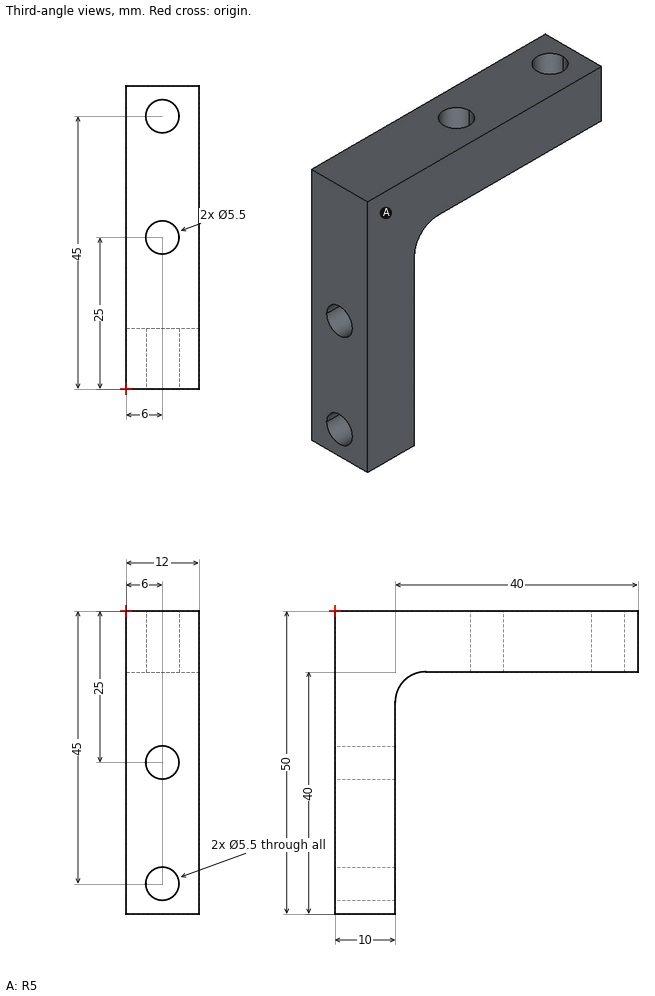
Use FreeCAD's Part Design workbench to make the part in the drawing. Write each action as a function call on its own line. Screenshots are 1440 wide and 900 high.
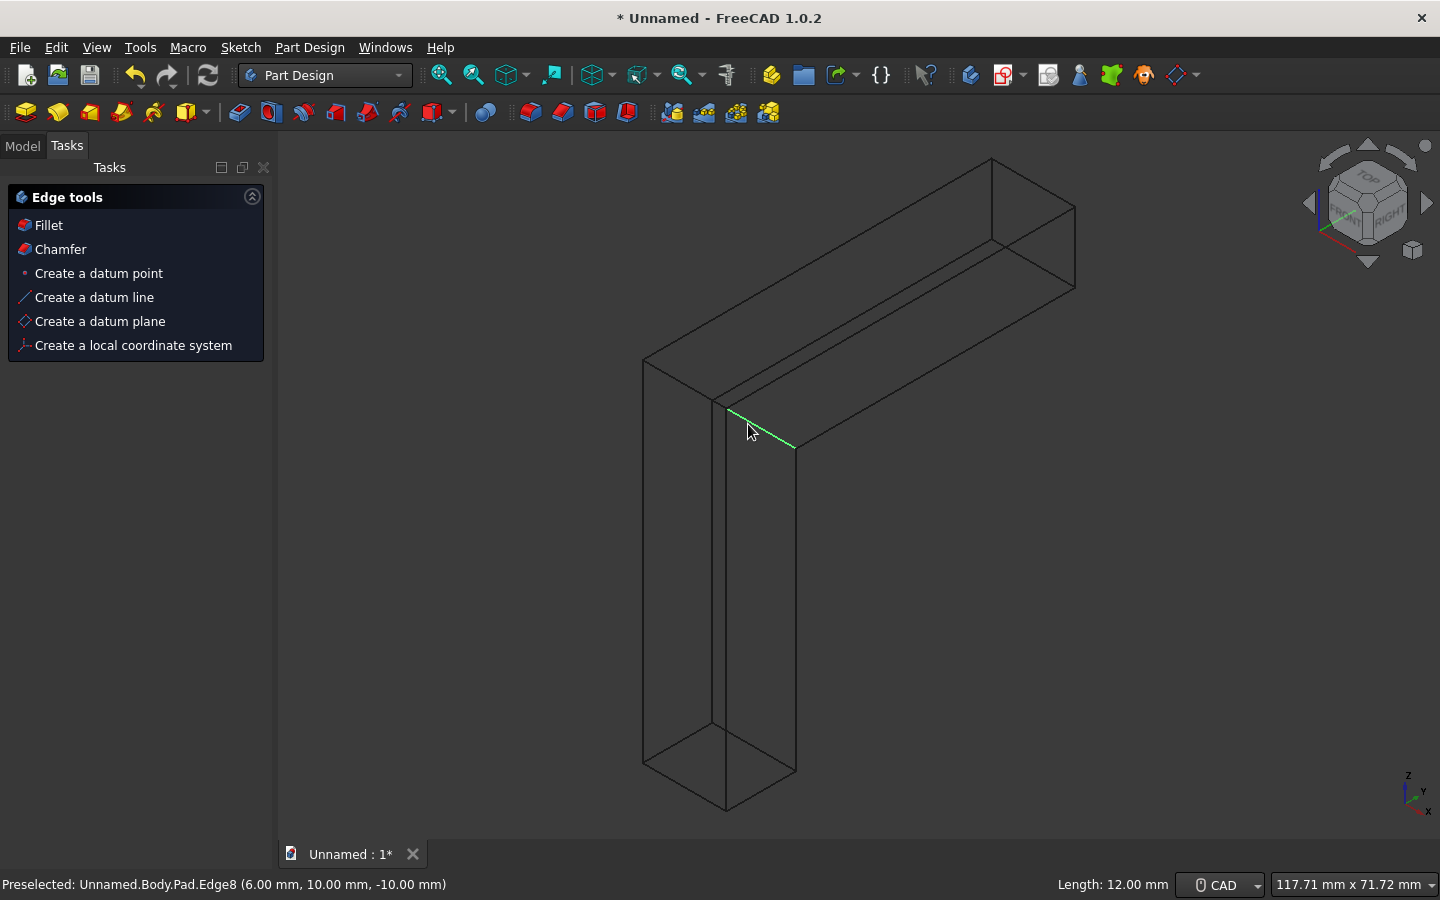
key(v)
key(1)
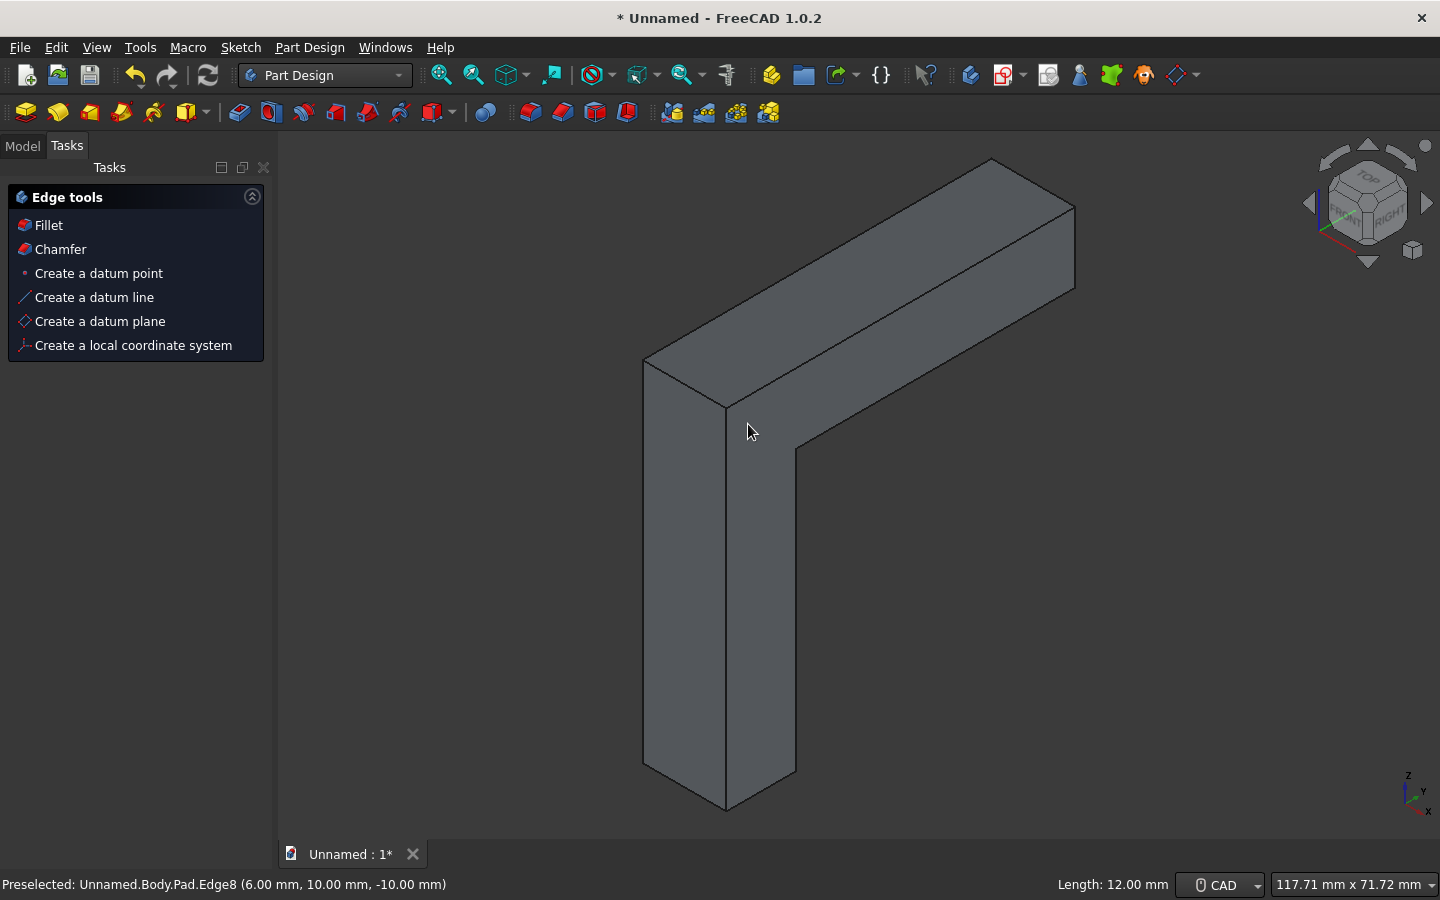
click(532, 112)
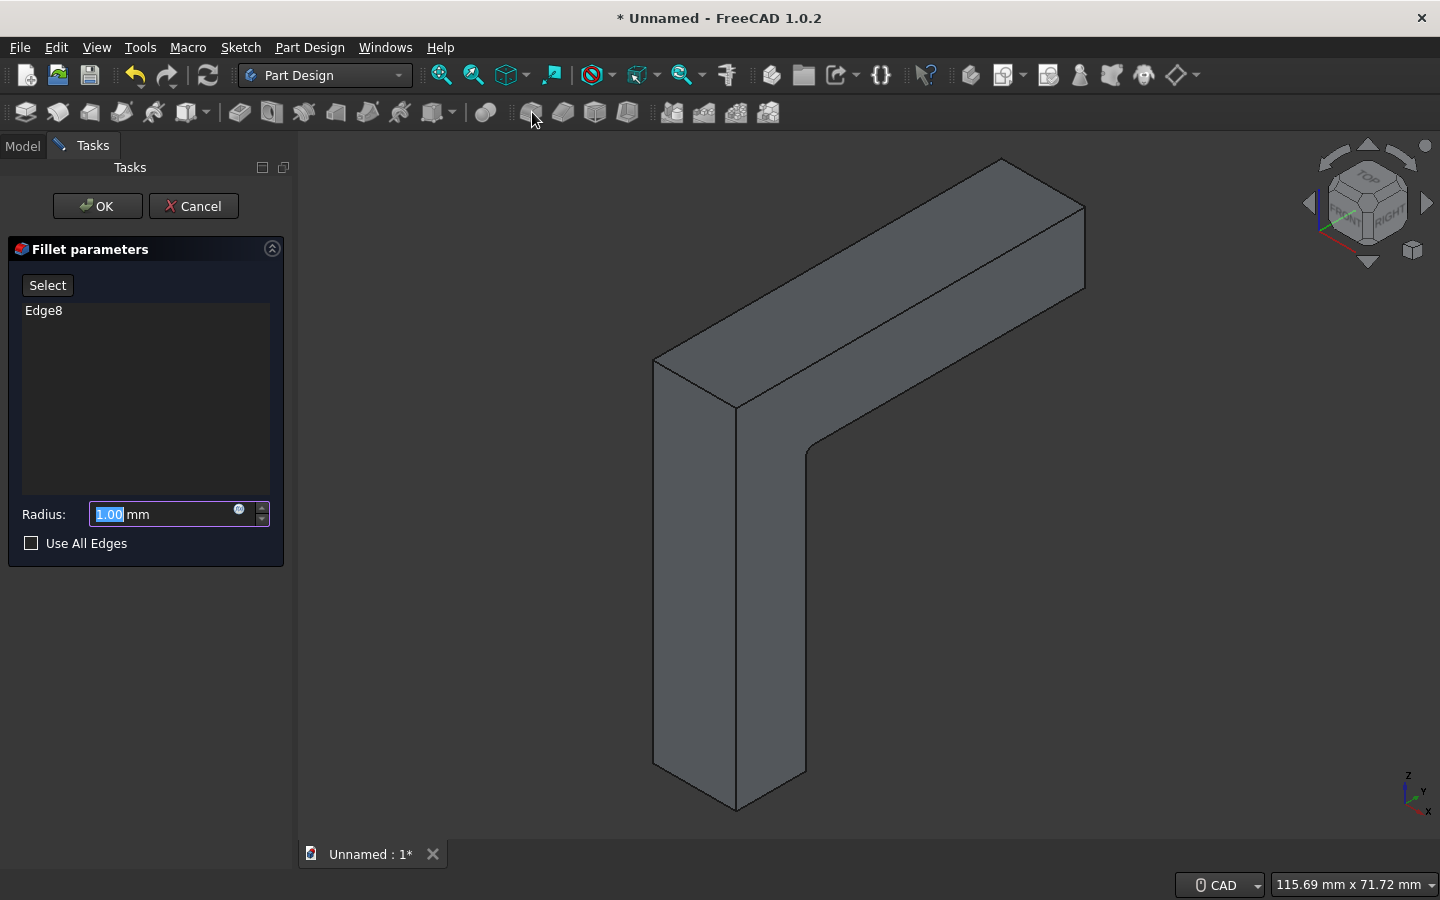
text(5)
key(Tab)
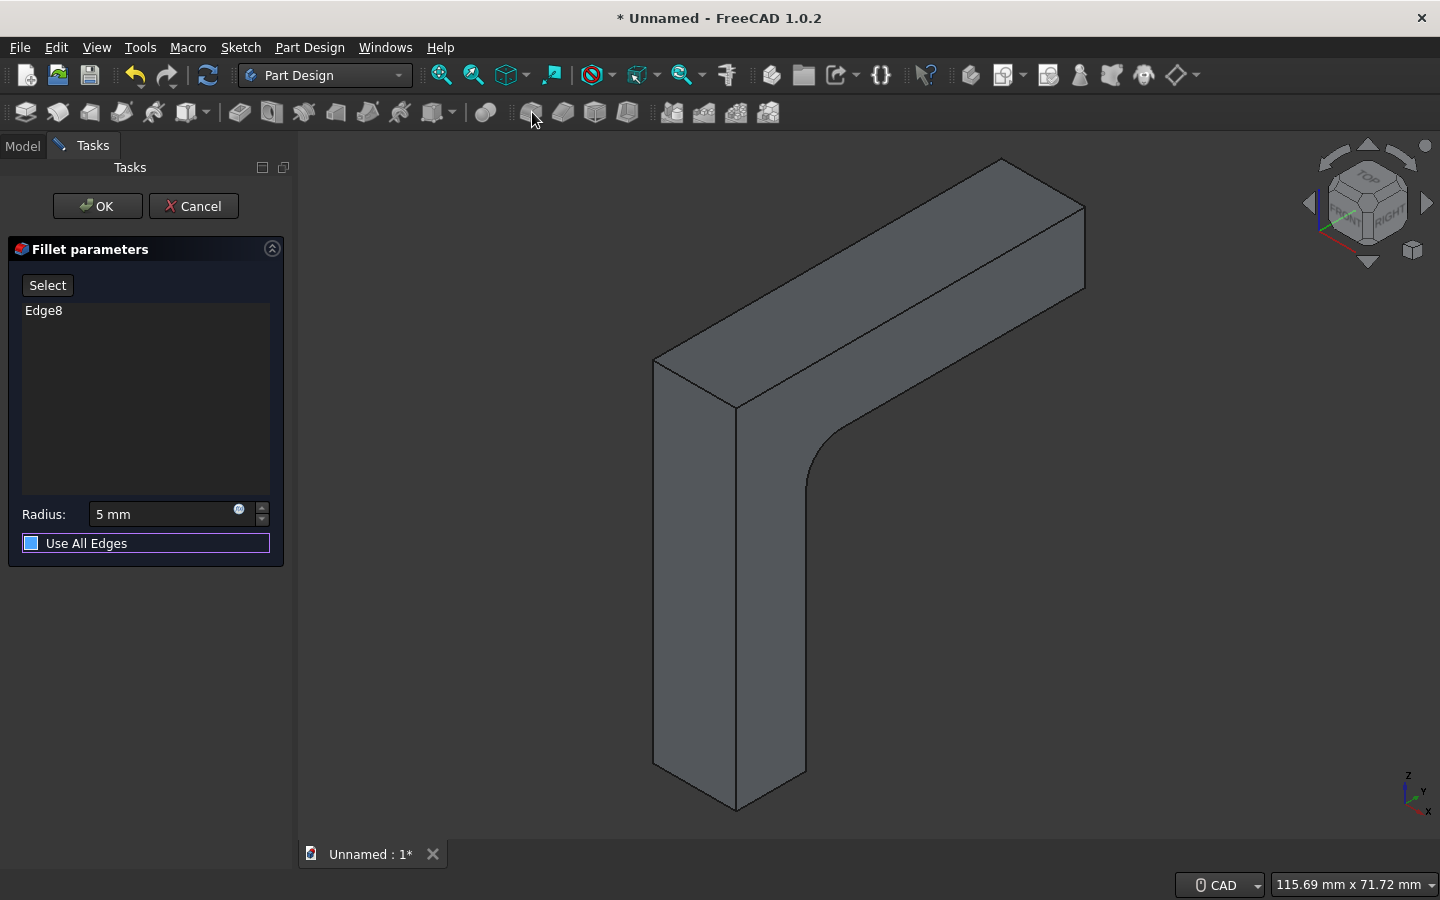
click(98, 206)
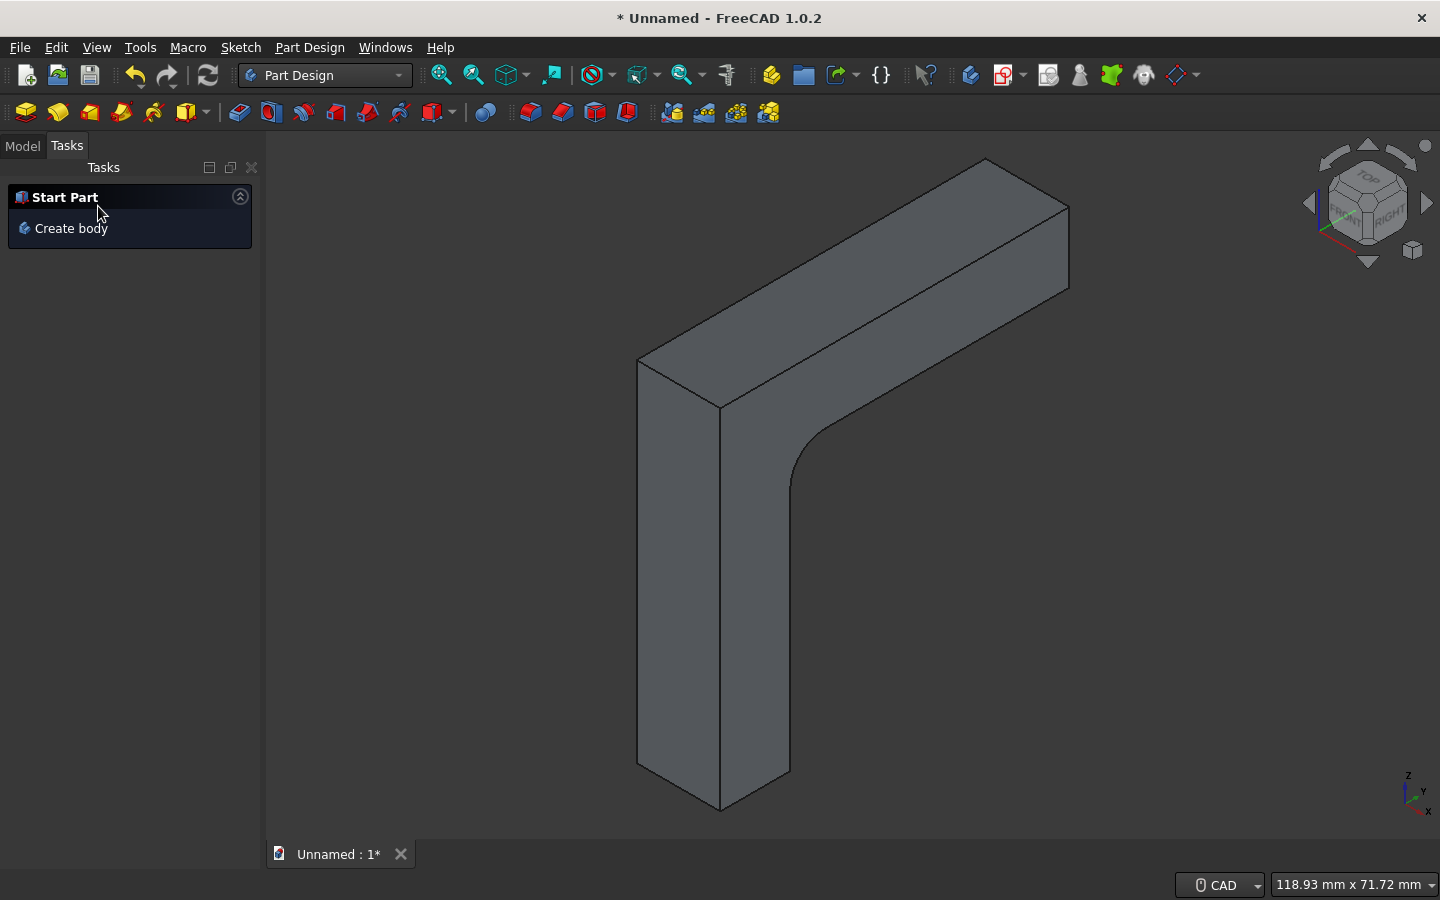
key(5)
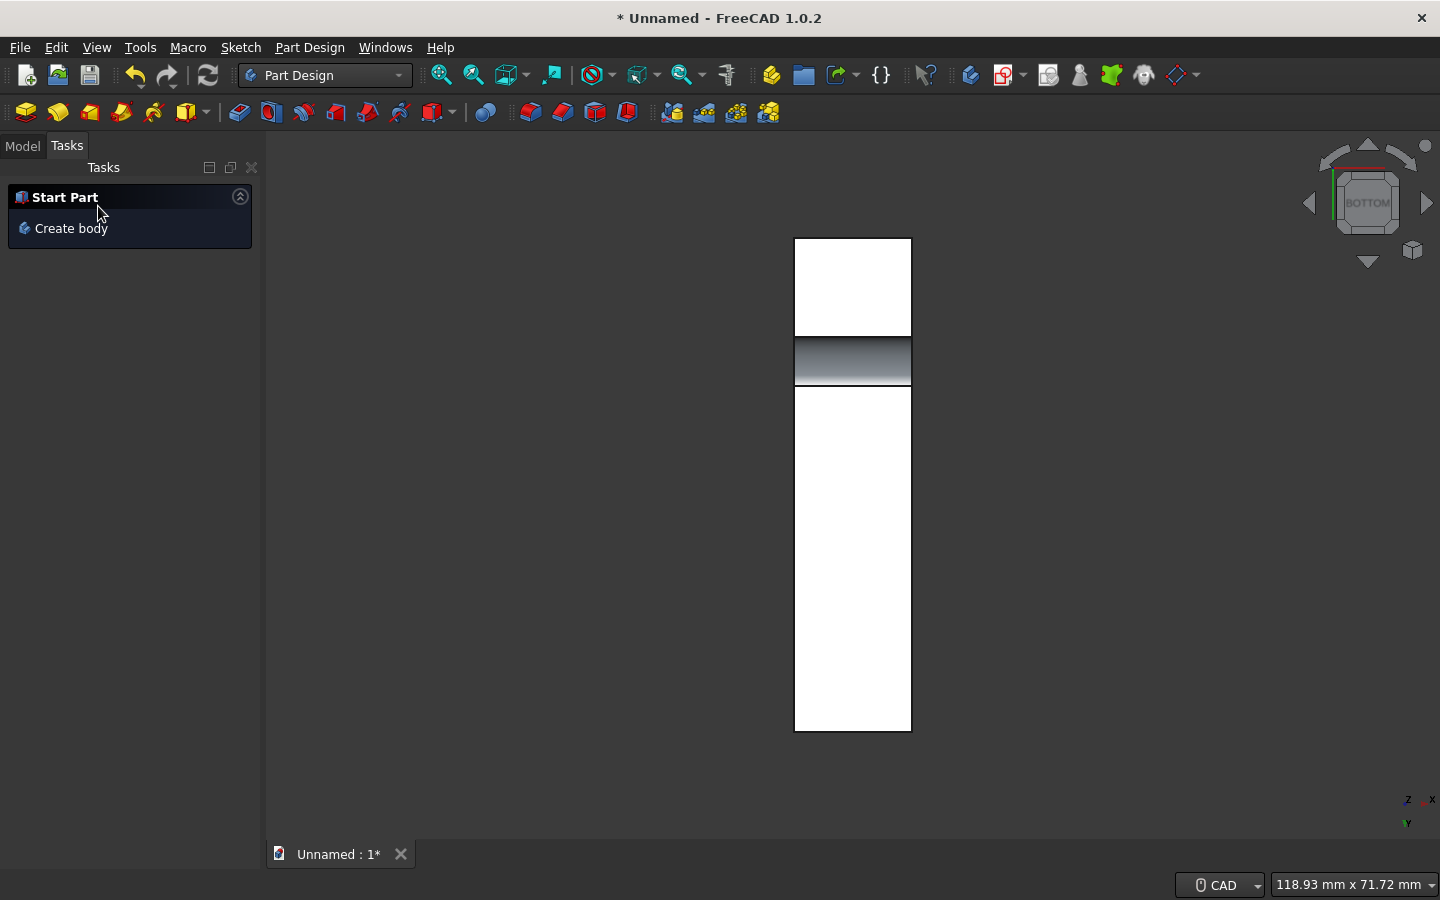
click(853, 657)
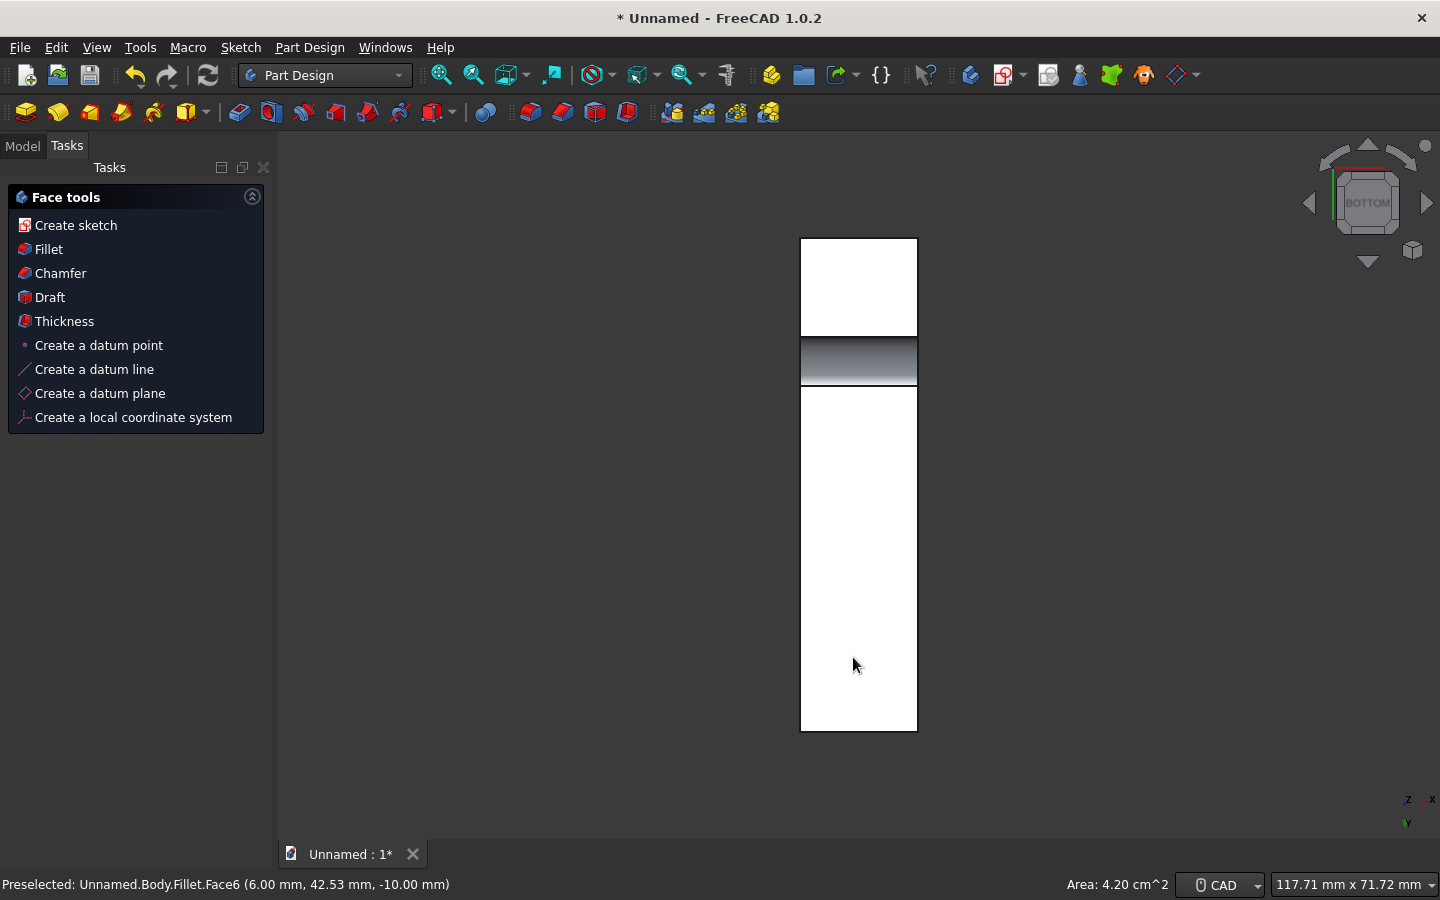
click(1004, 76)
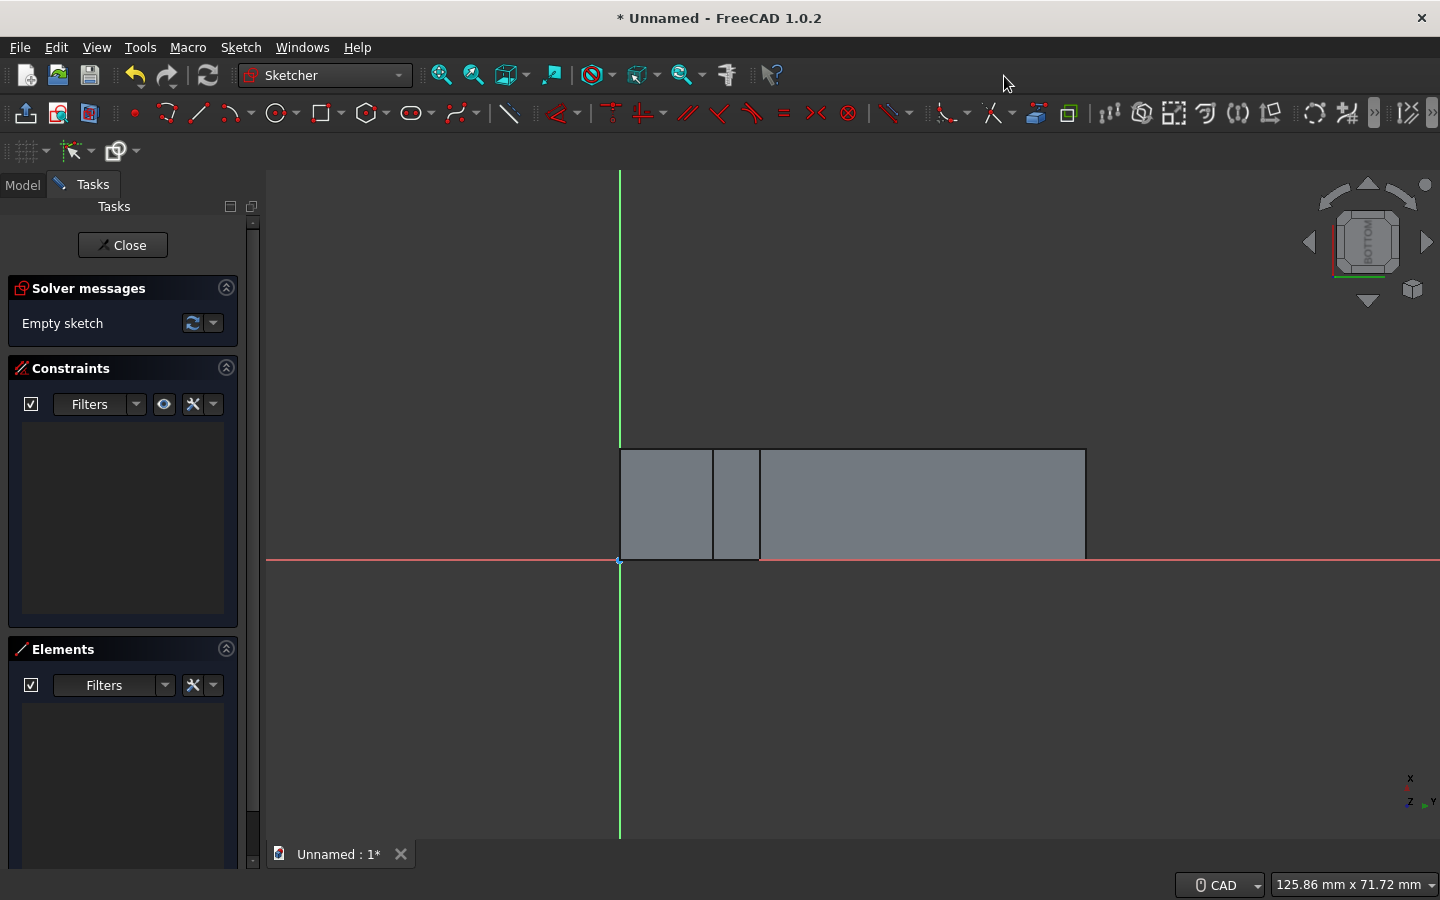
scroll(960, 550, up, 2)